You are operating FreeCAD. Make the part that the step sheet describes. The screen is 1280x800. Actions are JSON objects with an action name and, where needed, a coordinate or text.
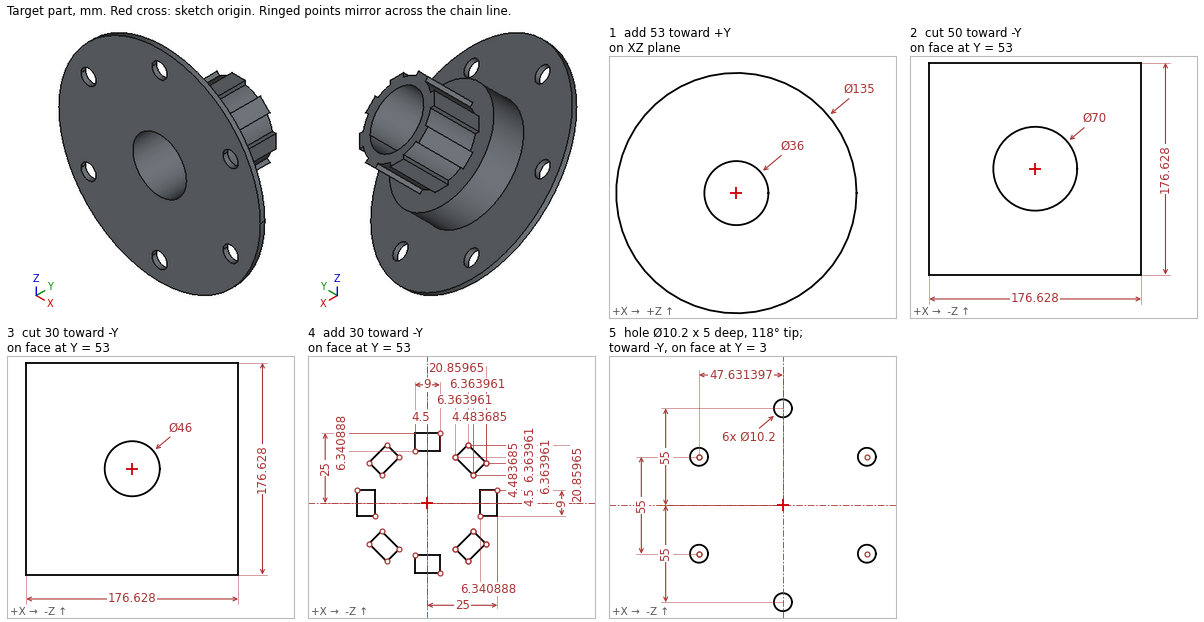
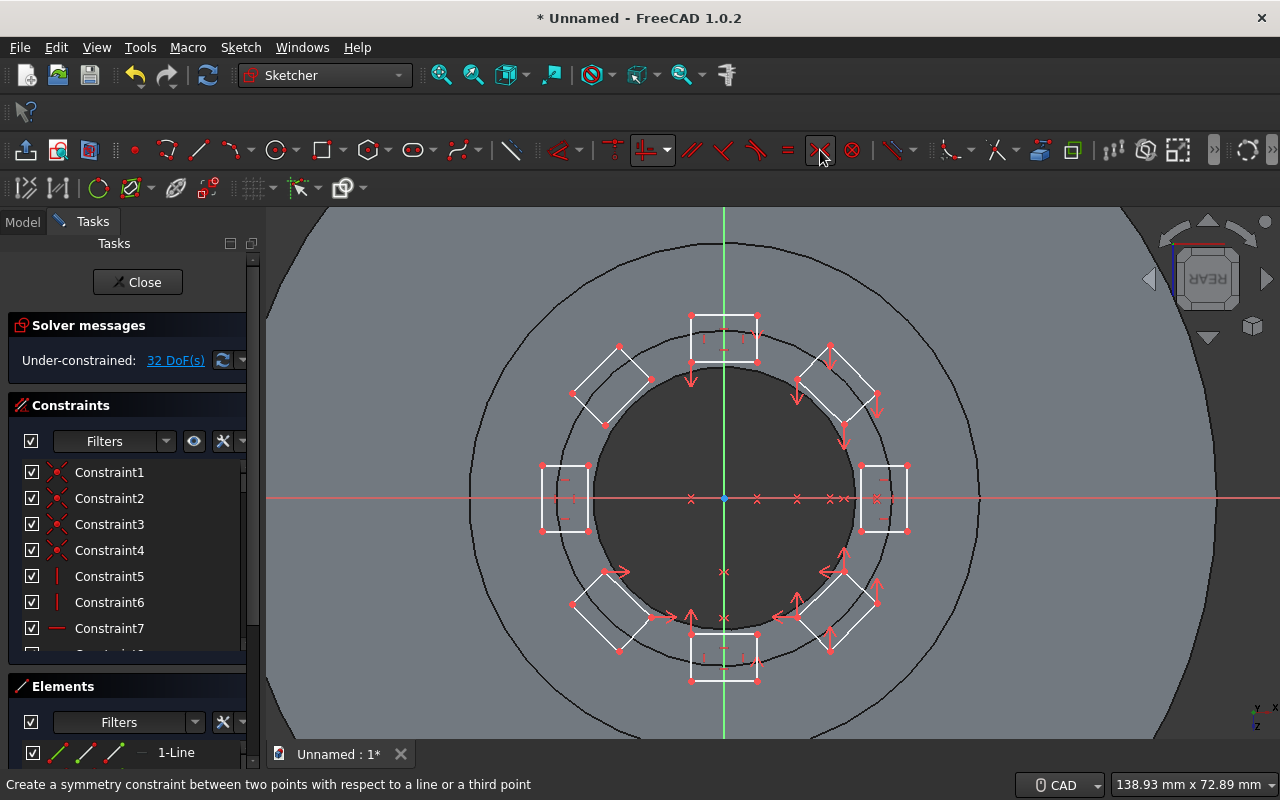
{"action": "left_click", "coordinate": [877, 603]}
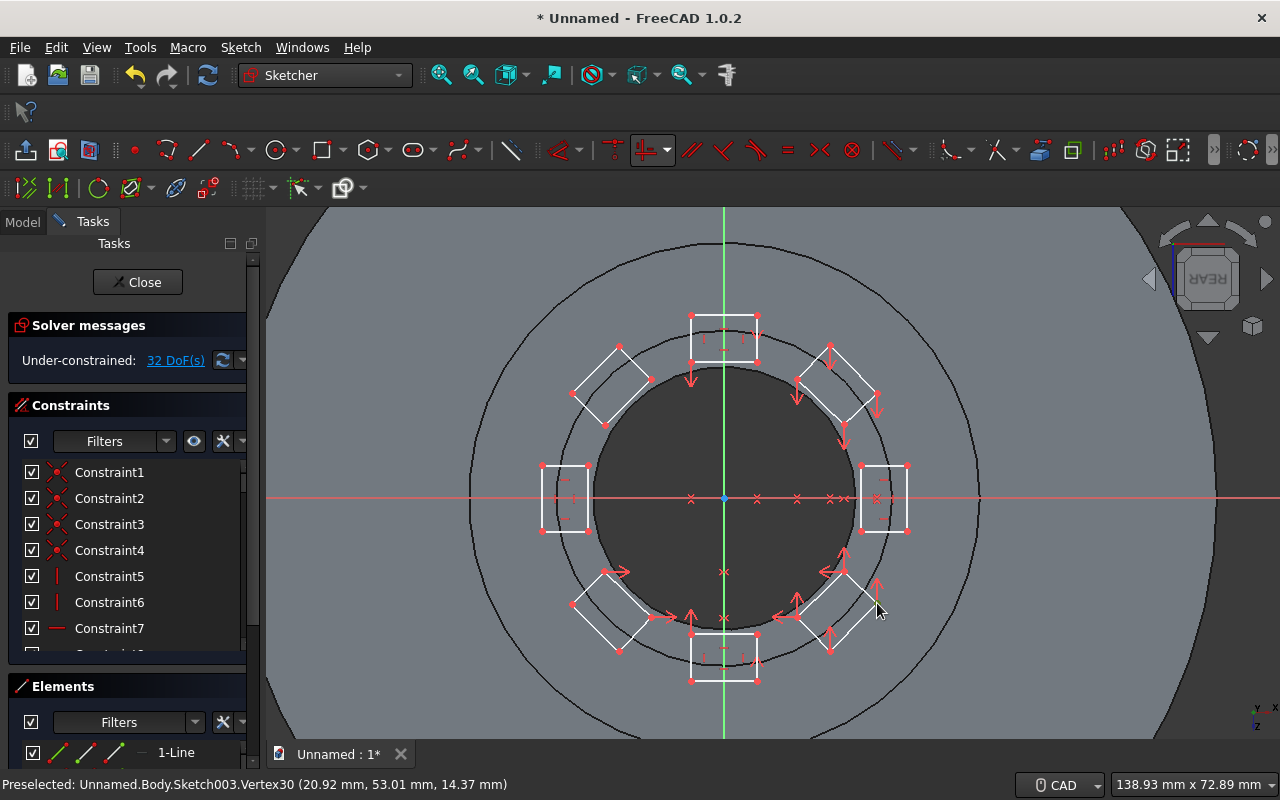
{"action": "left_click", "coordinate": [572, 605]}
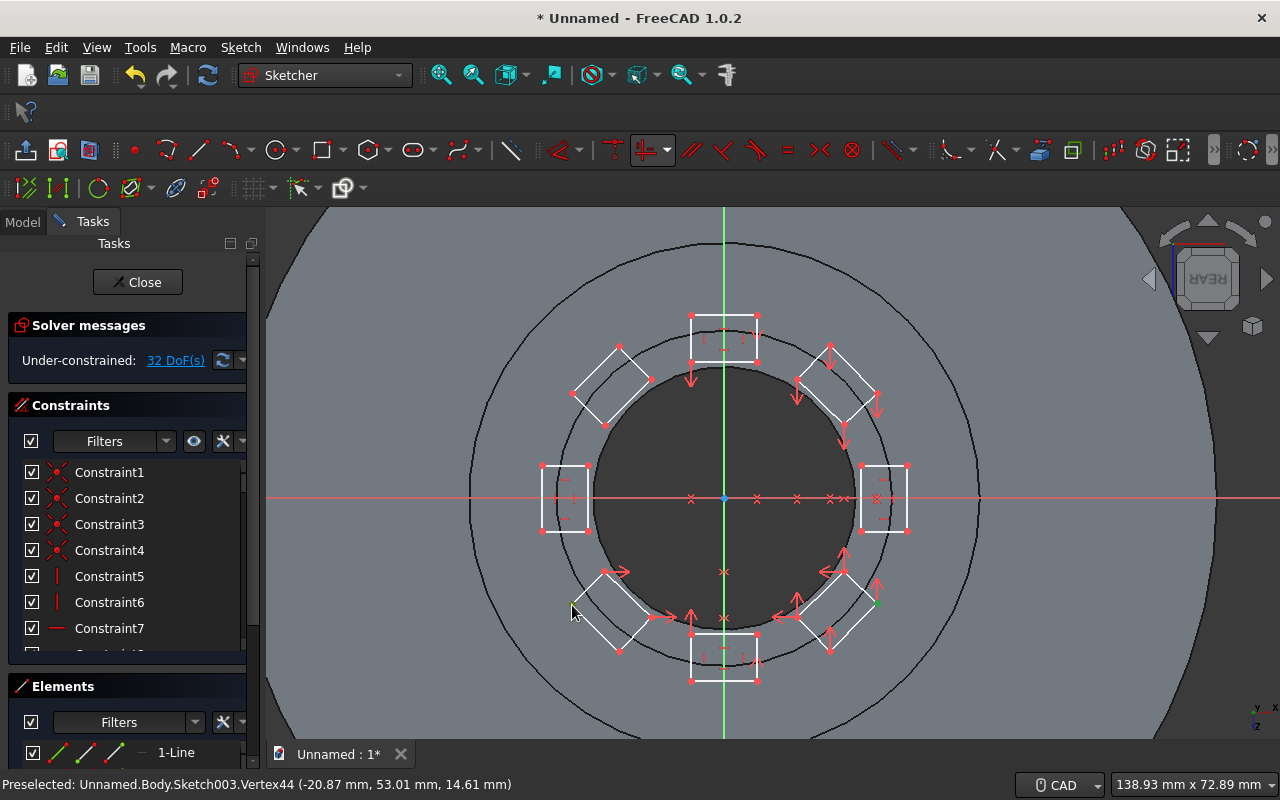
{"action": "left_click", "coordinate": [724, 541]}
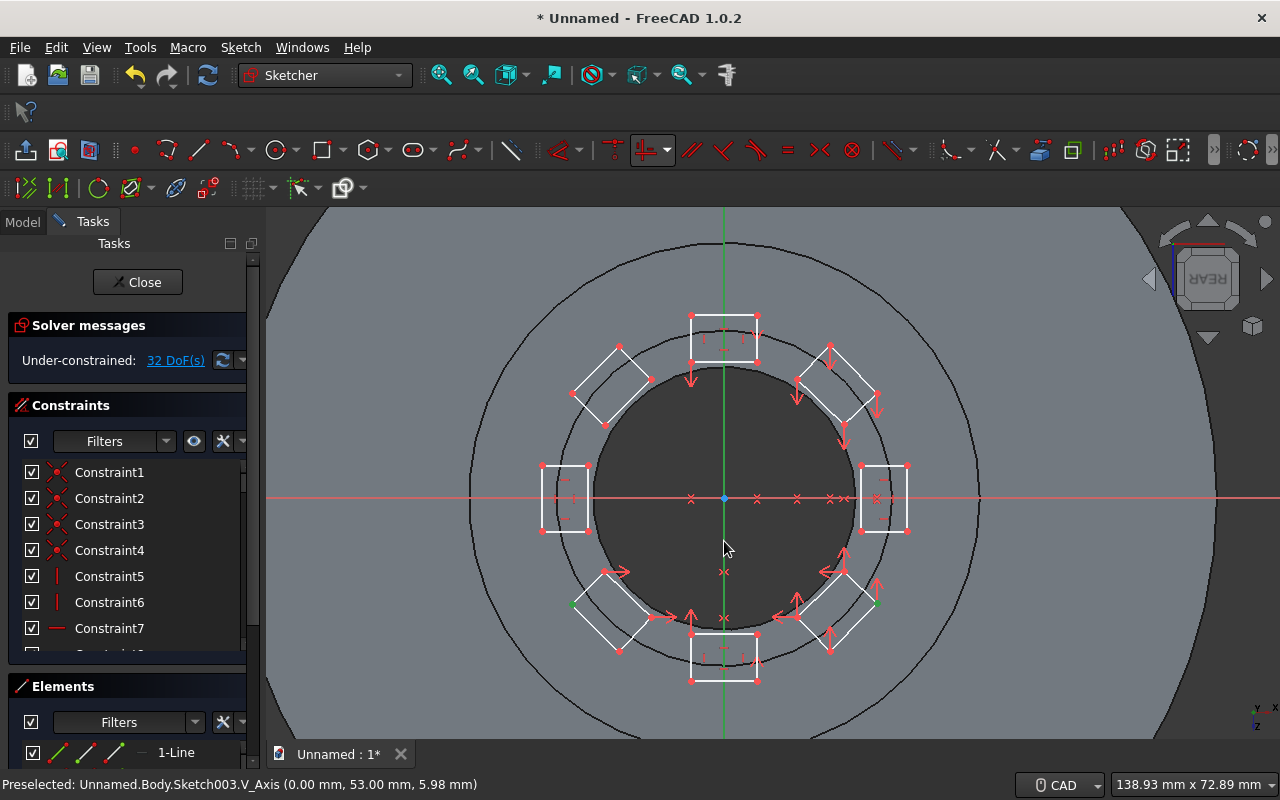
{"action": "left_click", "coordinate": [820, 150]}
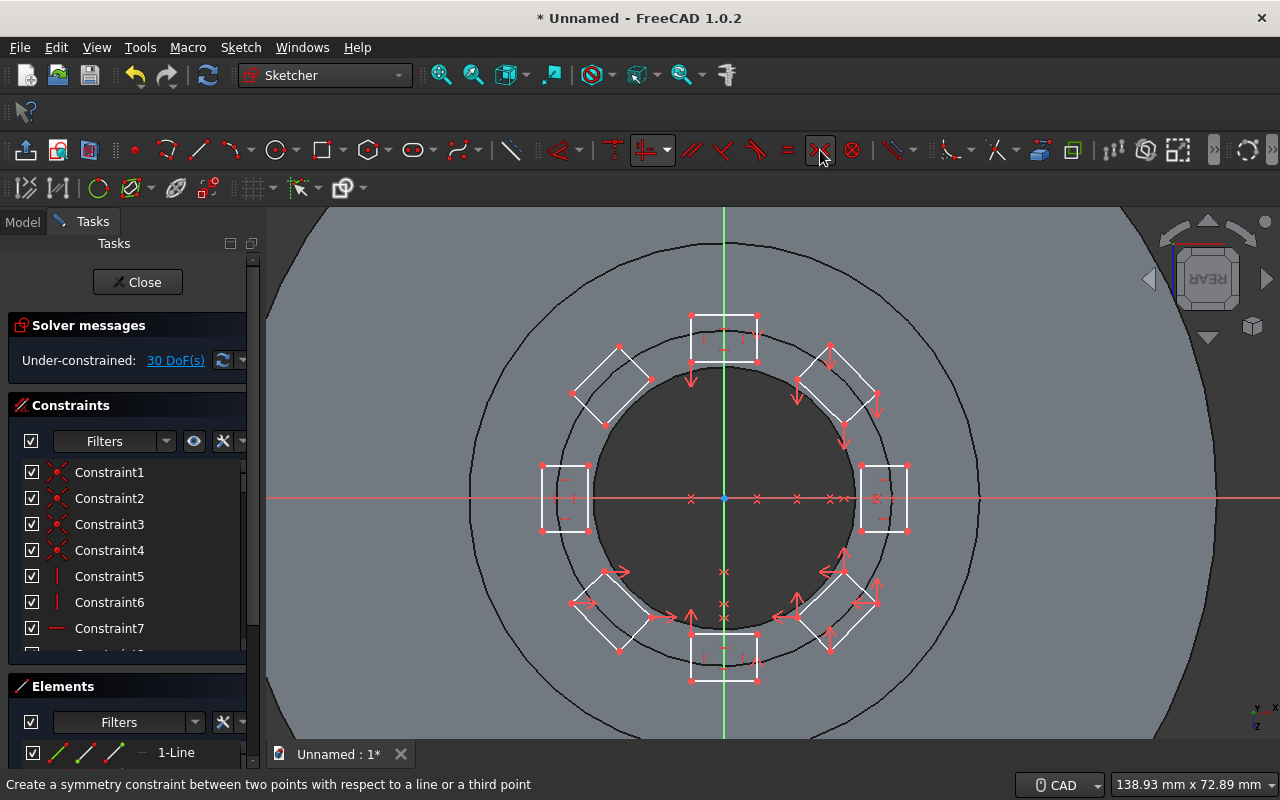
{"action": "left_click", "coordinate": [830, 651]}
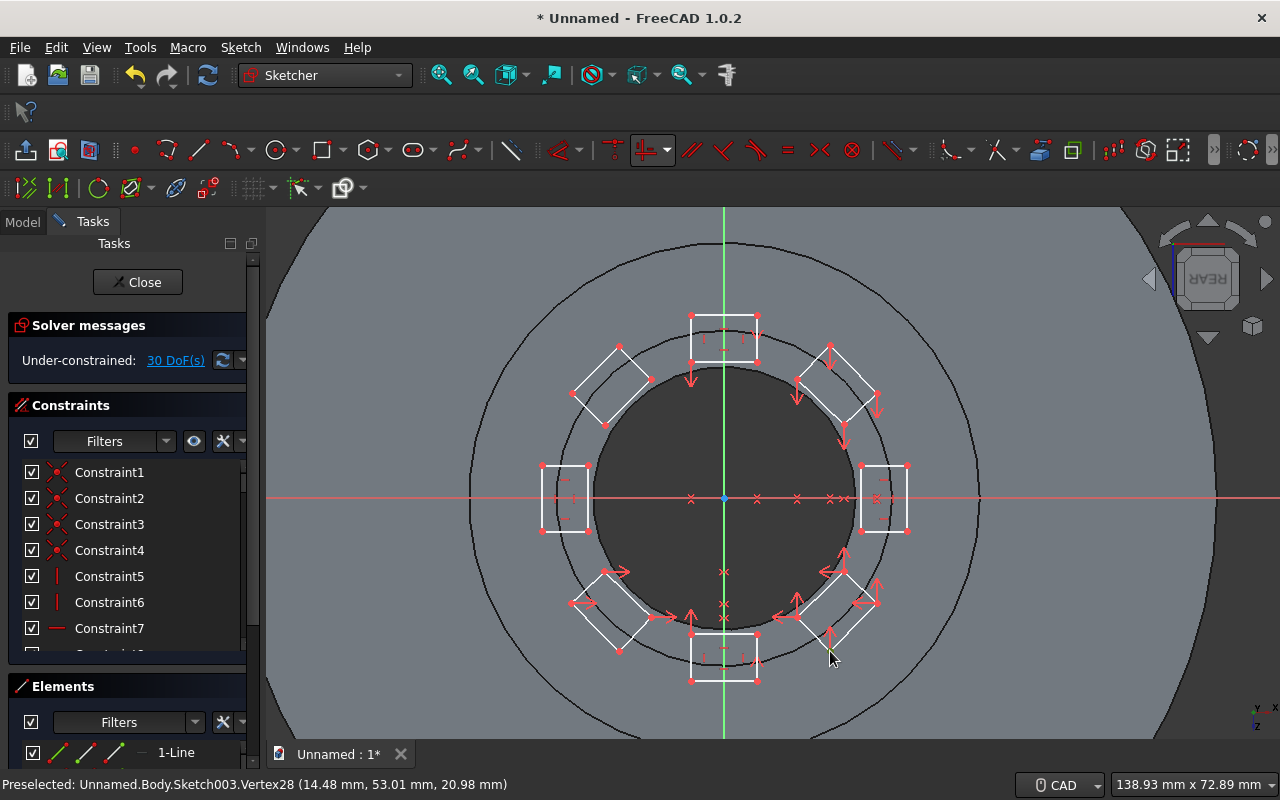
{"action": "left_click", "coordinate": [619, 652]}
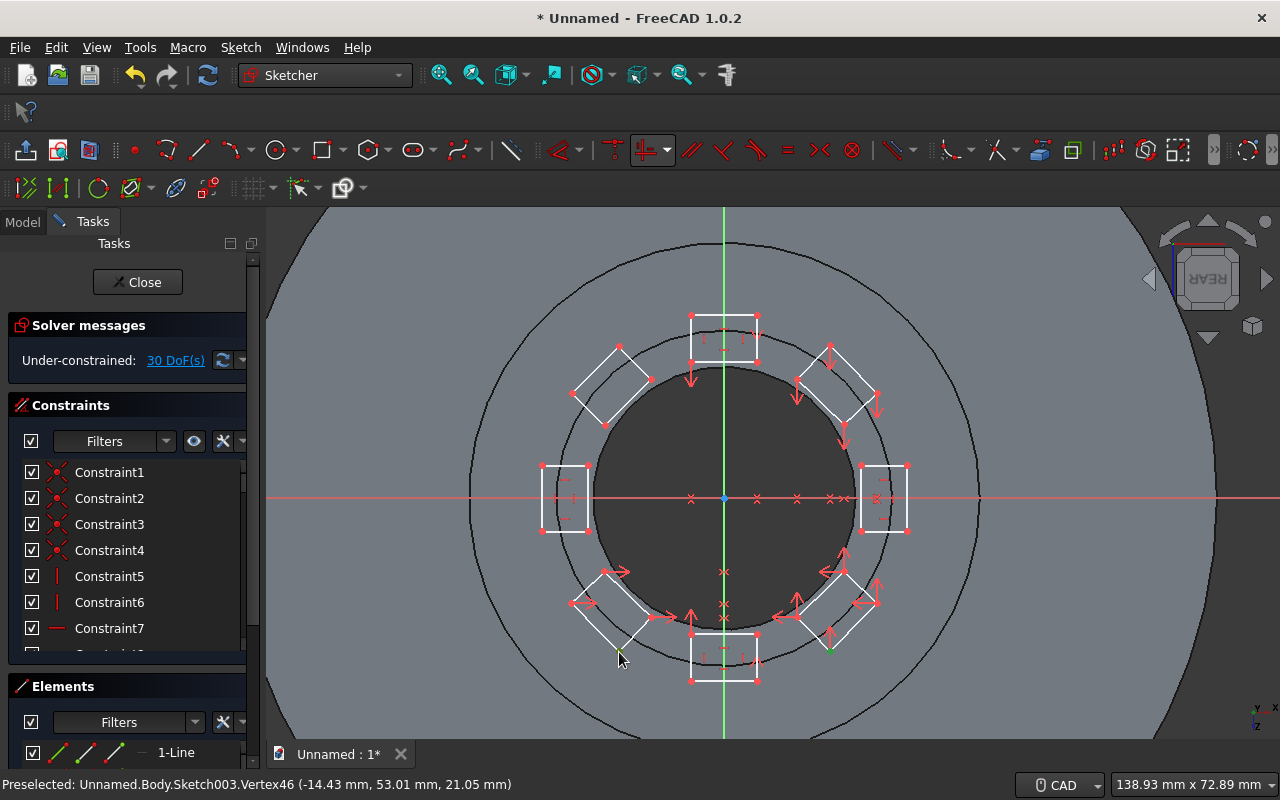
{"action": "left_click", "coordinate": [724, 541]}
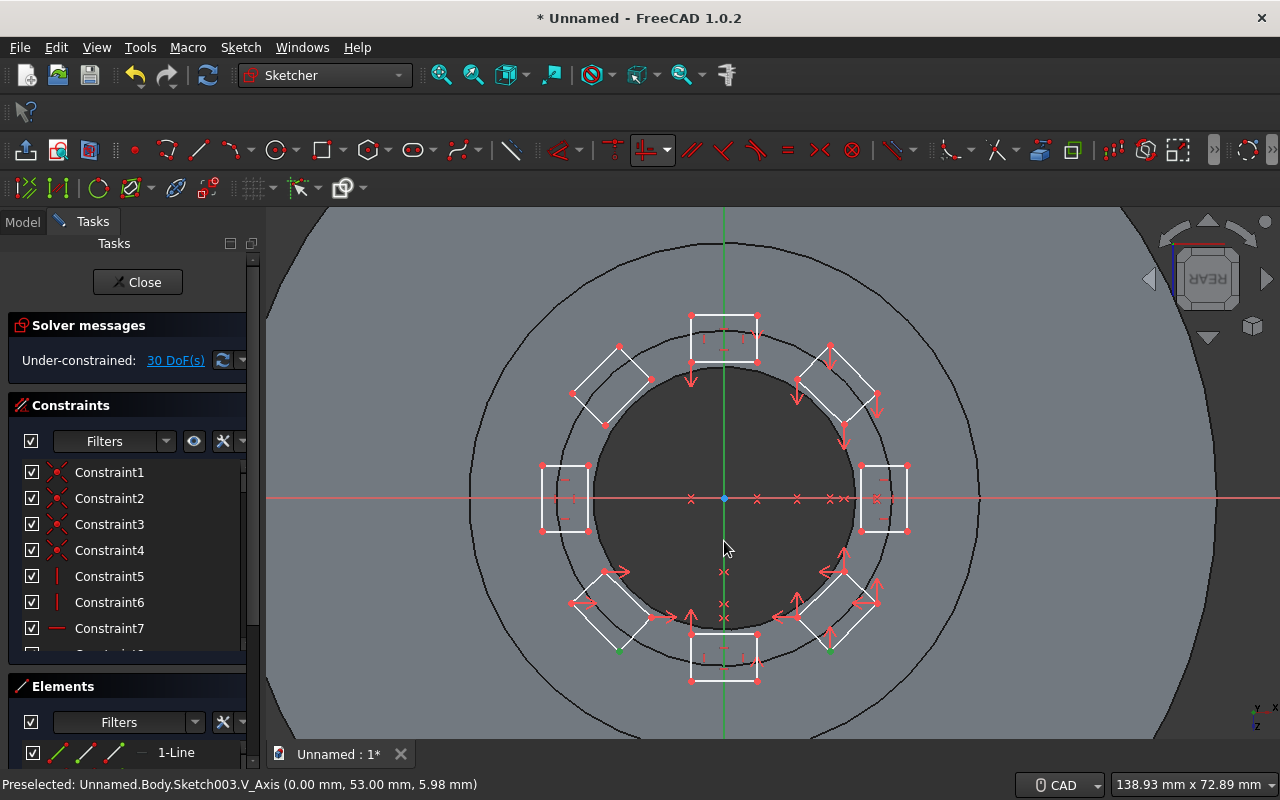
{"action": "left_click", "coordinate": [820, 150]}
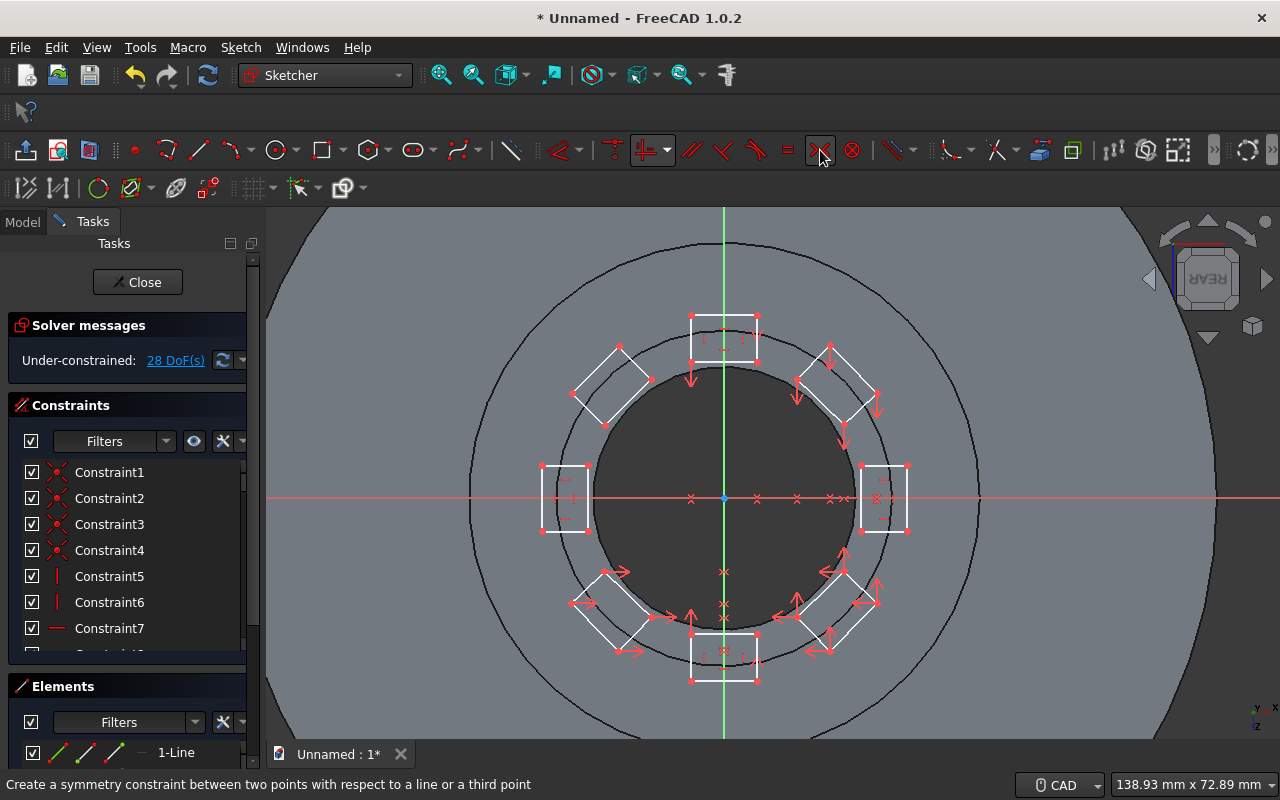
{"action": "left_click", "coordinate": [907, 466]}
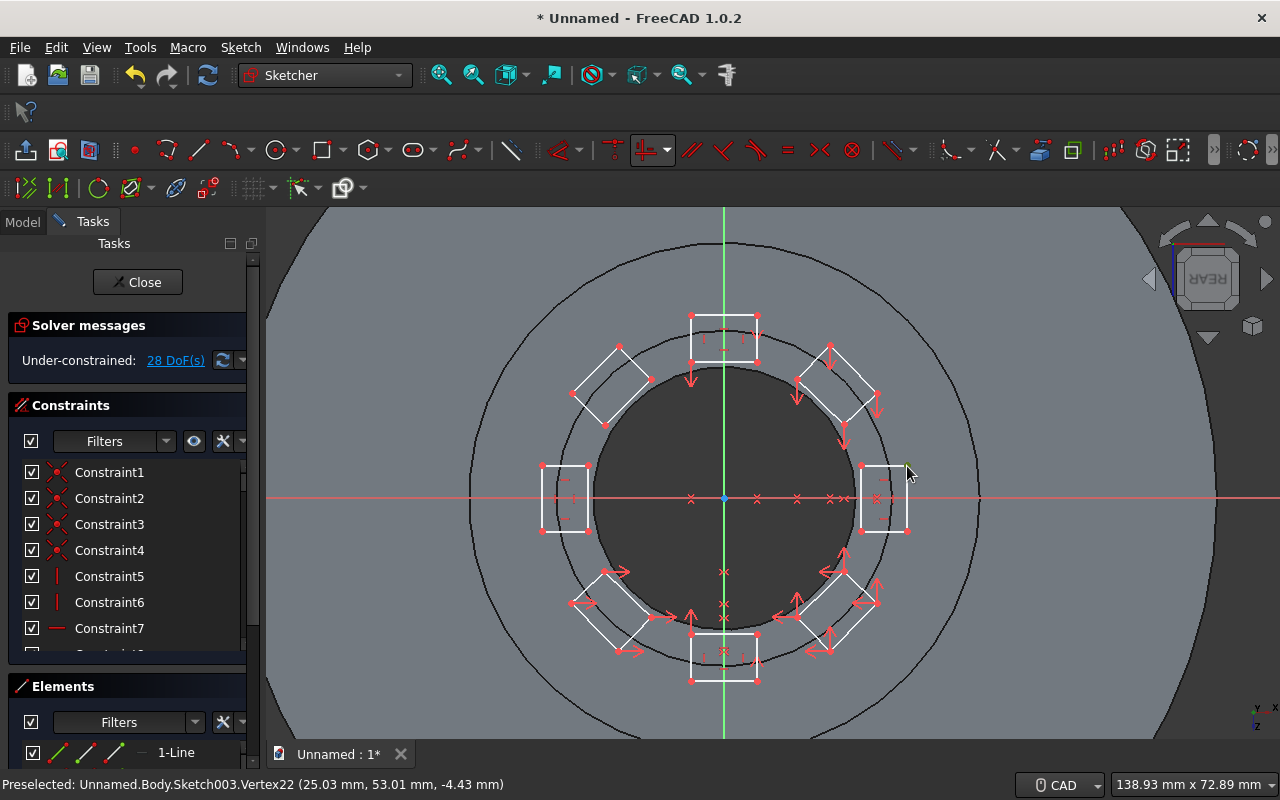
{"action": "left_click", "coordinate": [542, 466]}